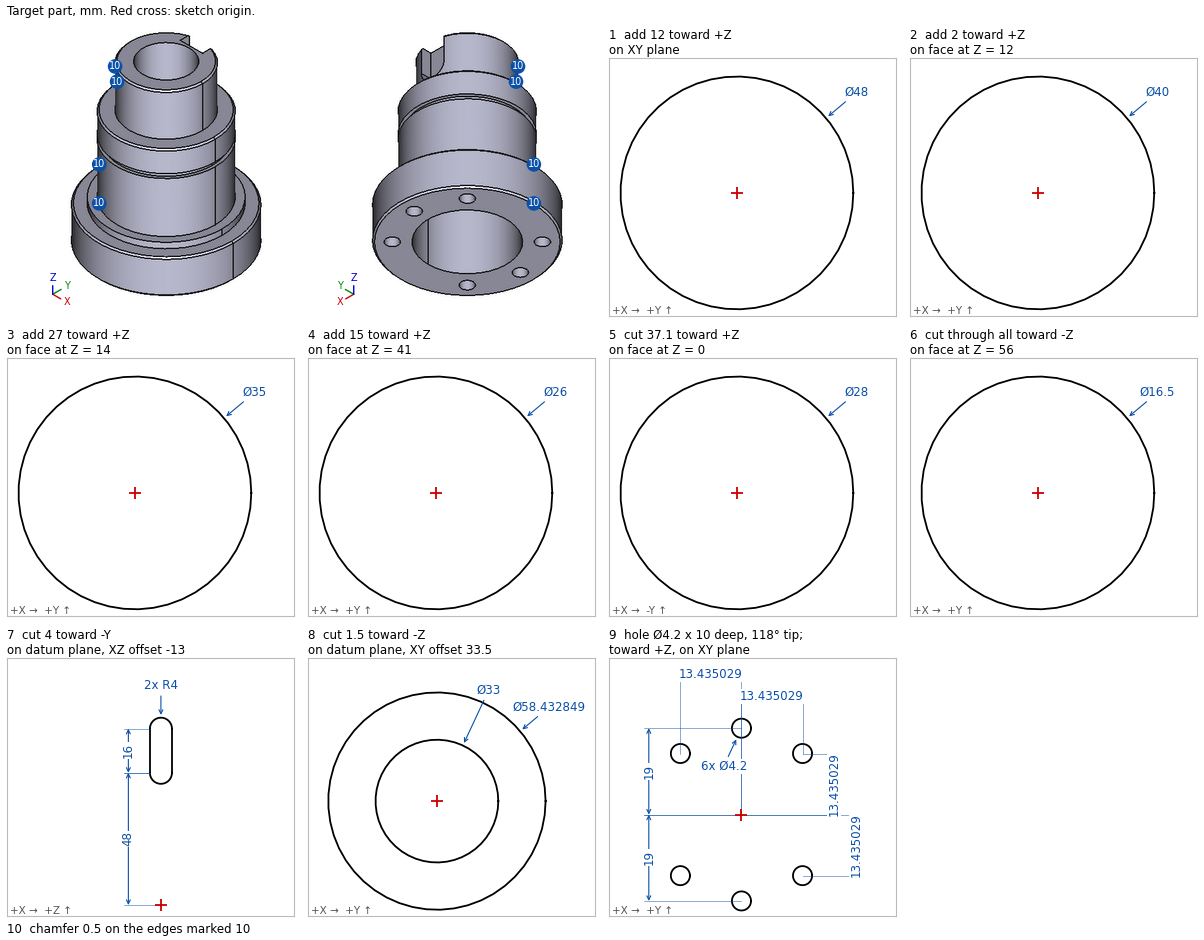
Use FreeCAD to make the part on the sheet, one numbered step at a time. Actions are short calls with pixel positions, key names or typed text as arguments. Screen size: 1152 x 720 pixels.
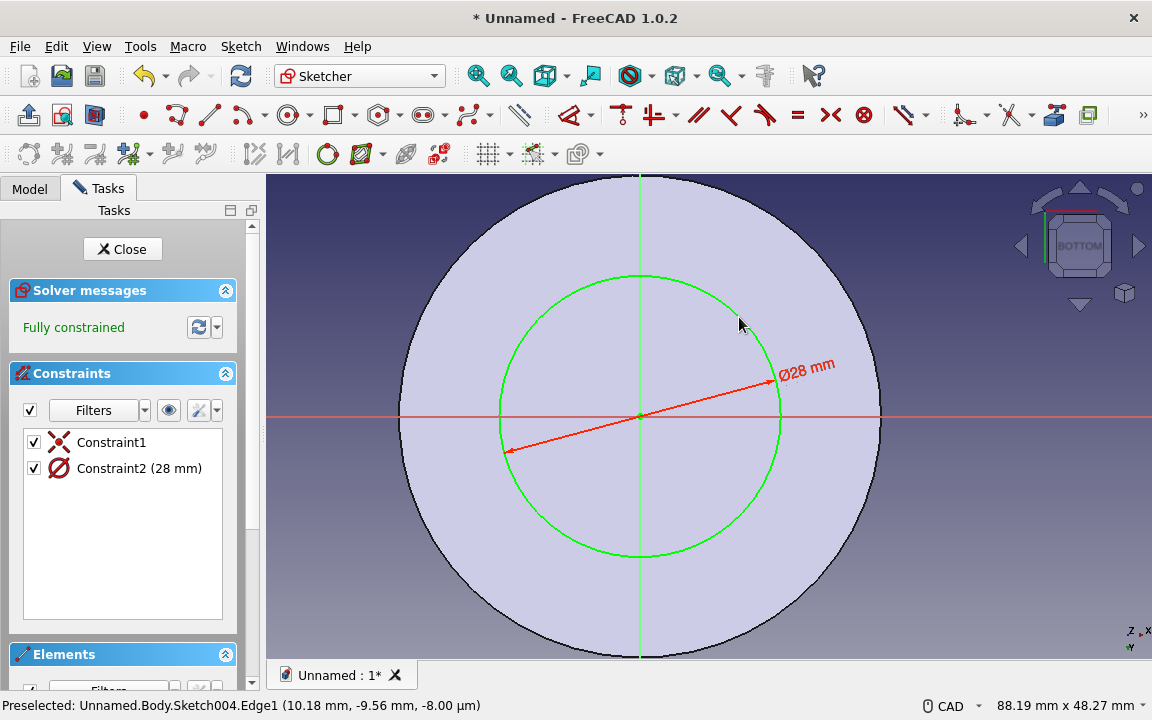
click(123, 249)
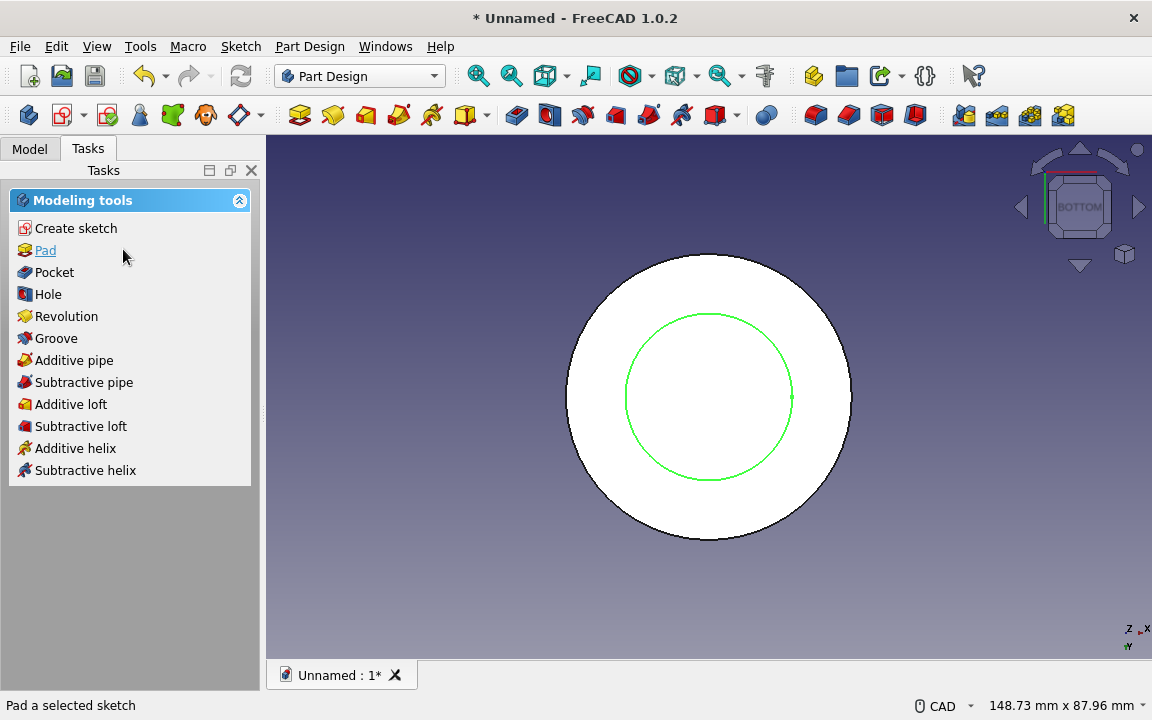
click(517, 116)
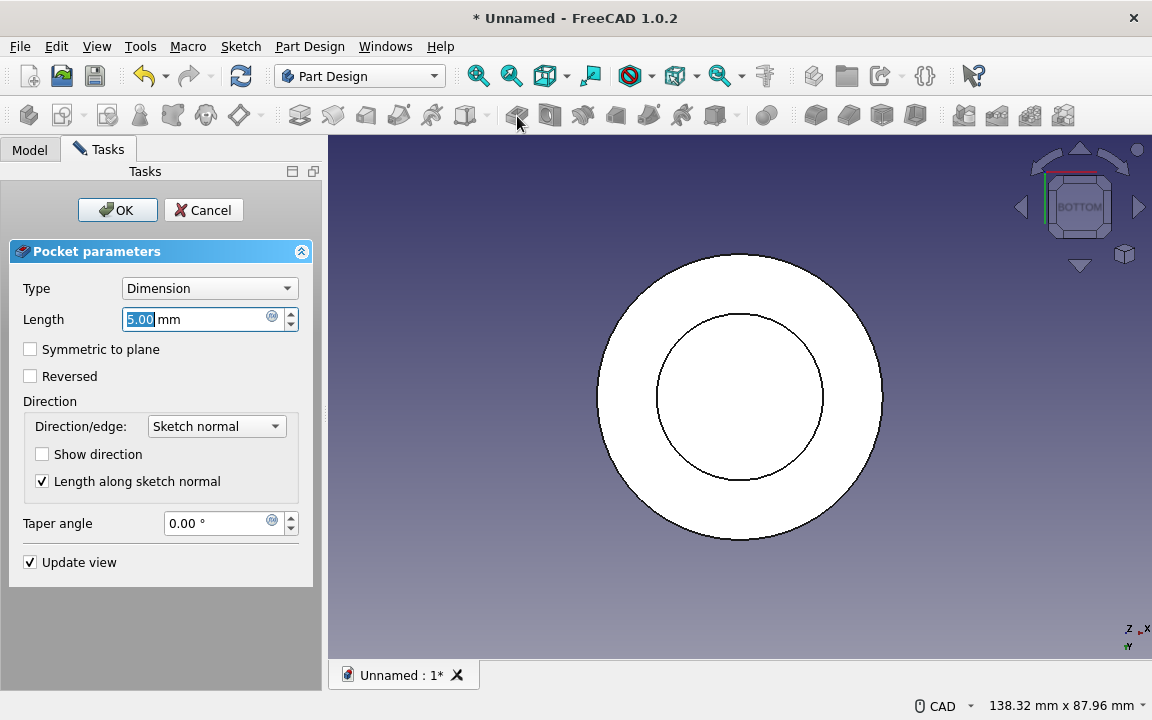
text(37.1)
key(Tab)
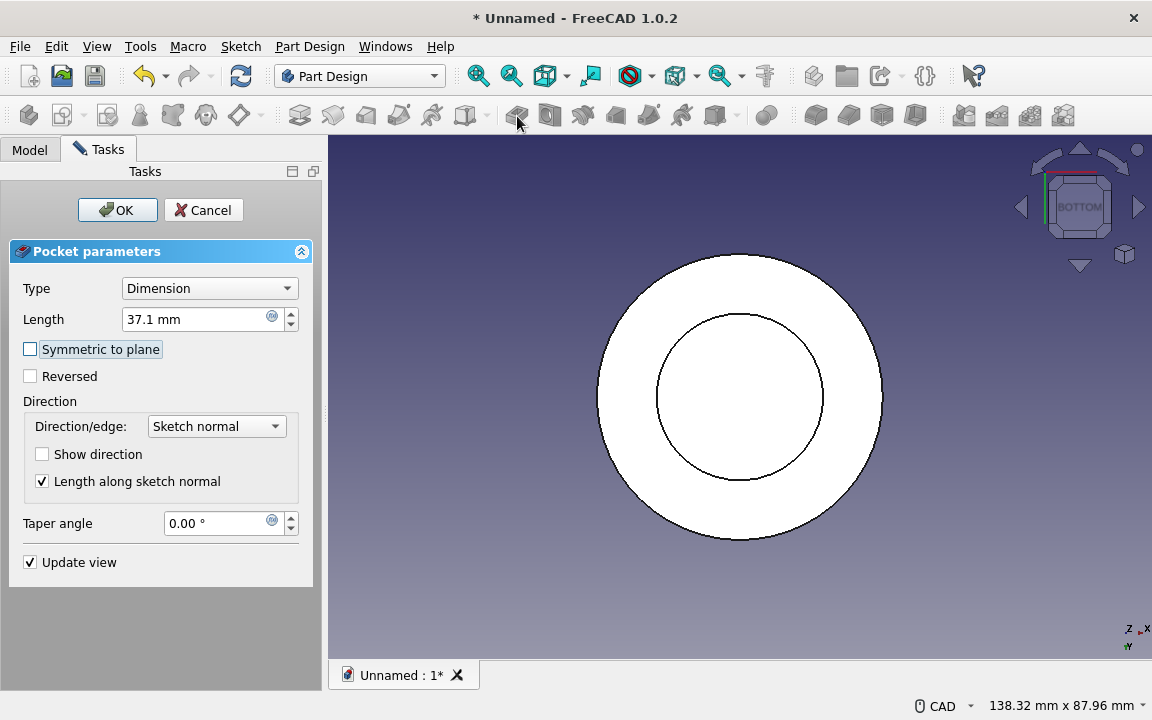
click(118, 210)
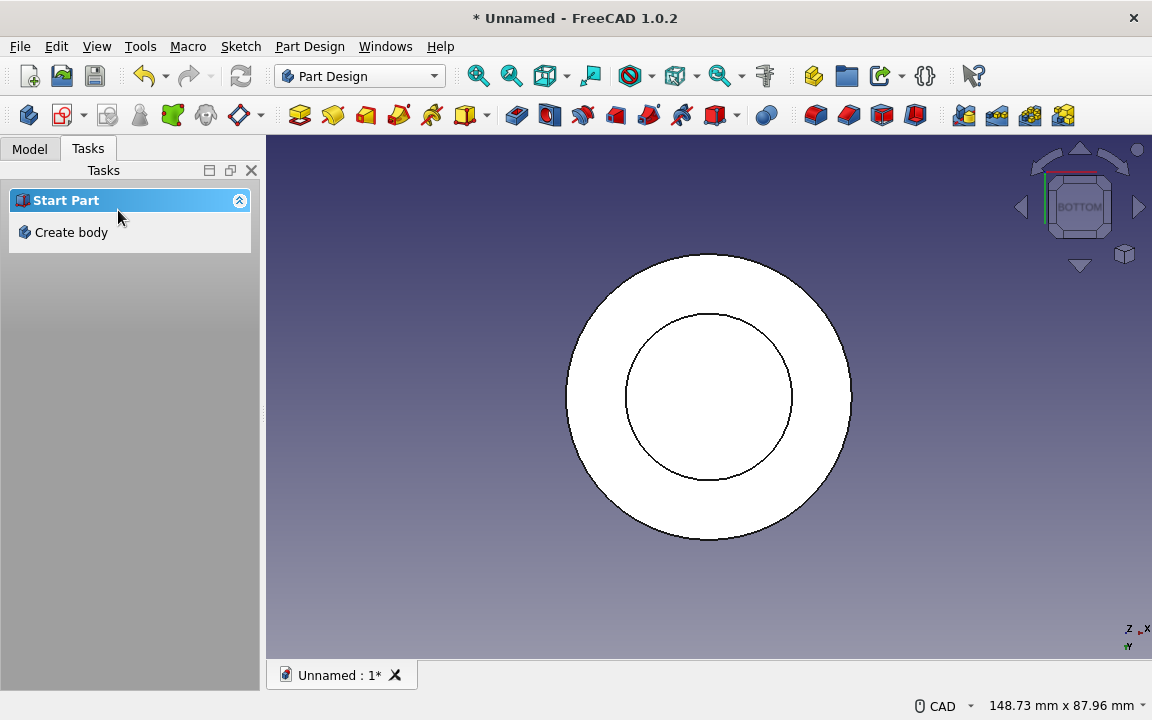
key(0)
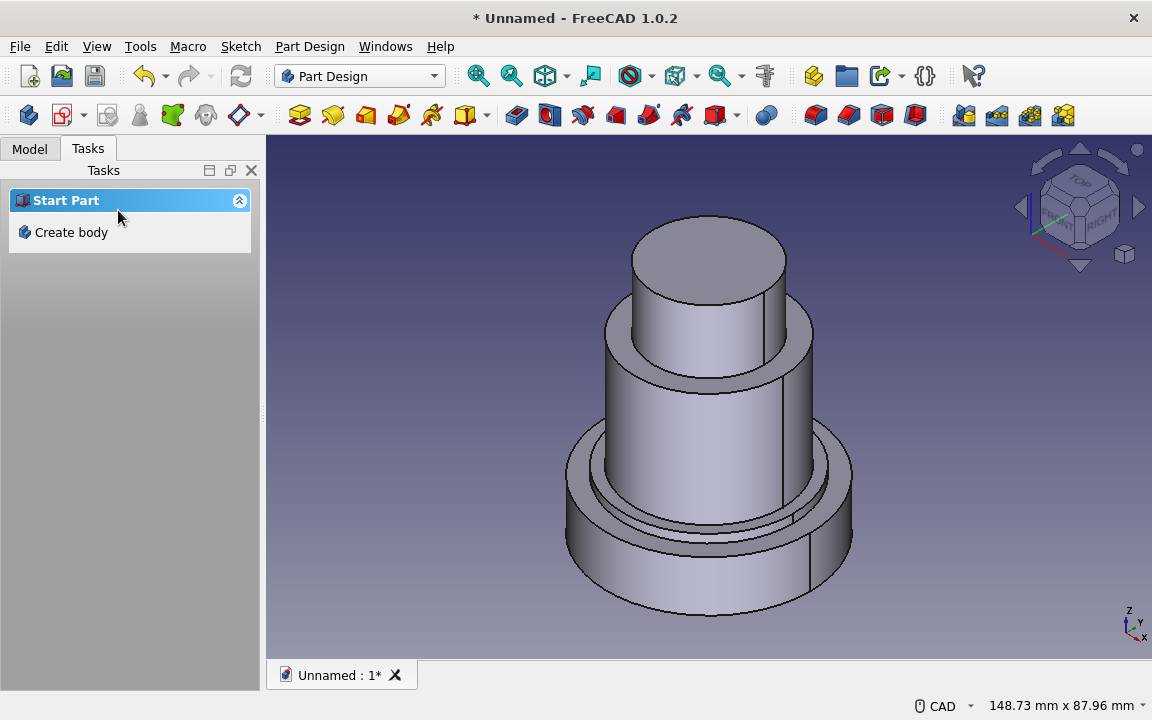
click(709, 260)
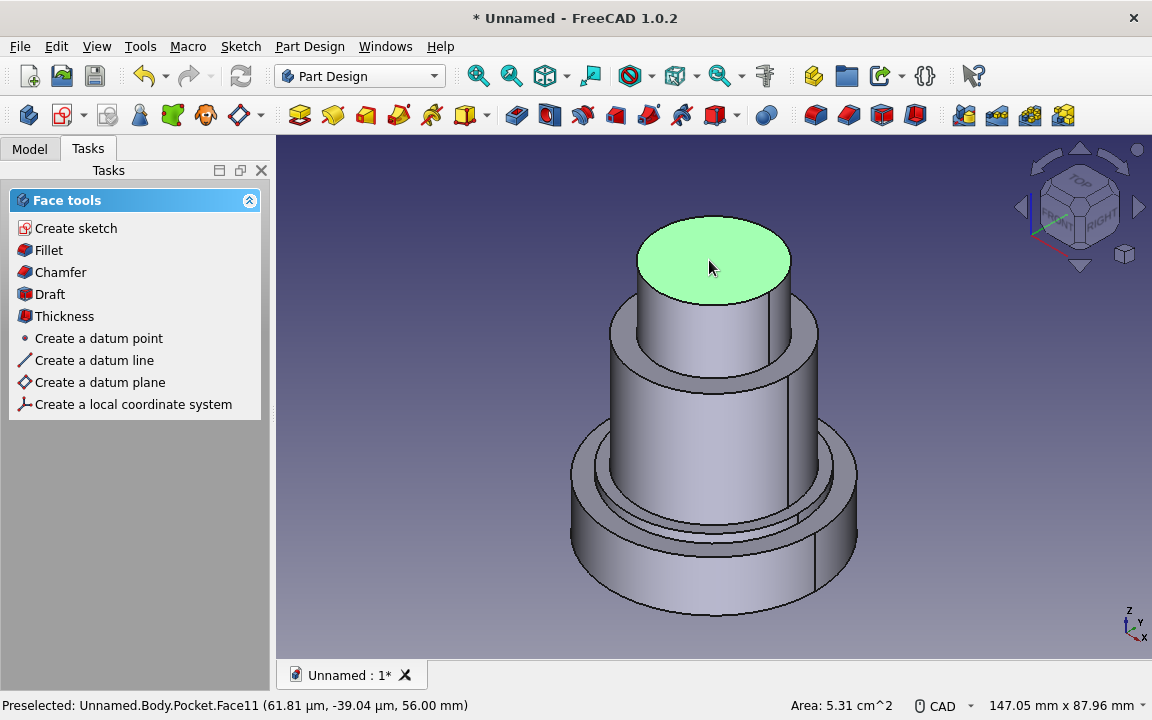
click(62, 116)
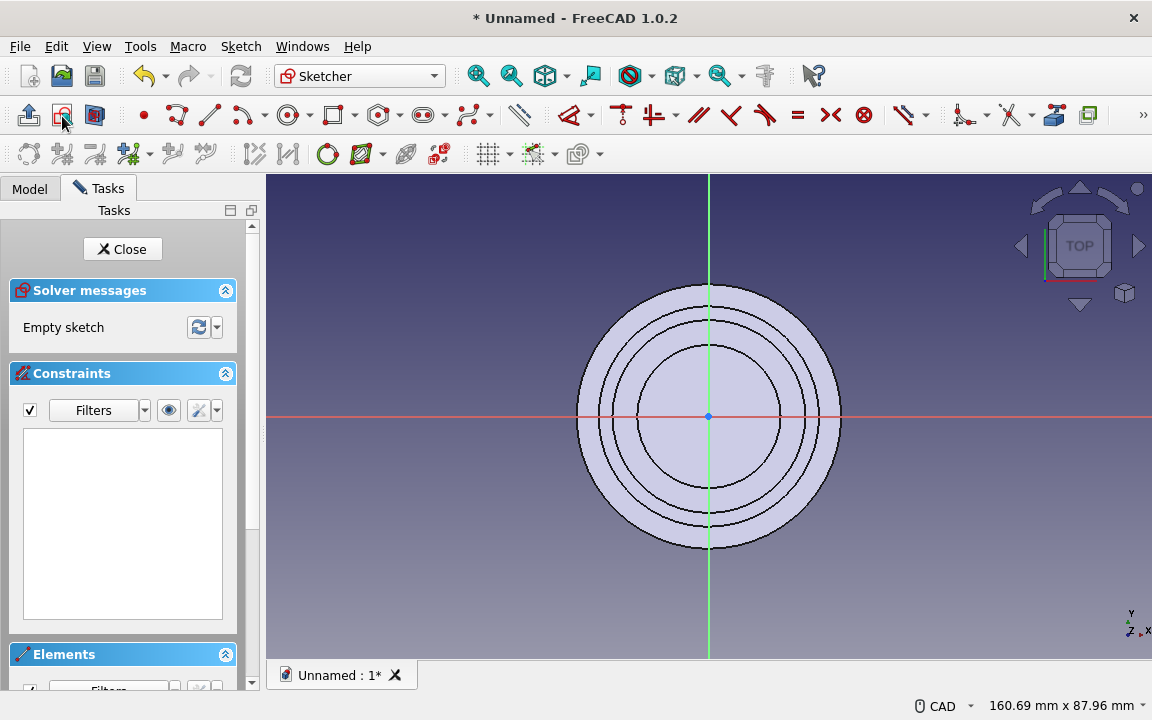
scroll(738, 416, up, 6)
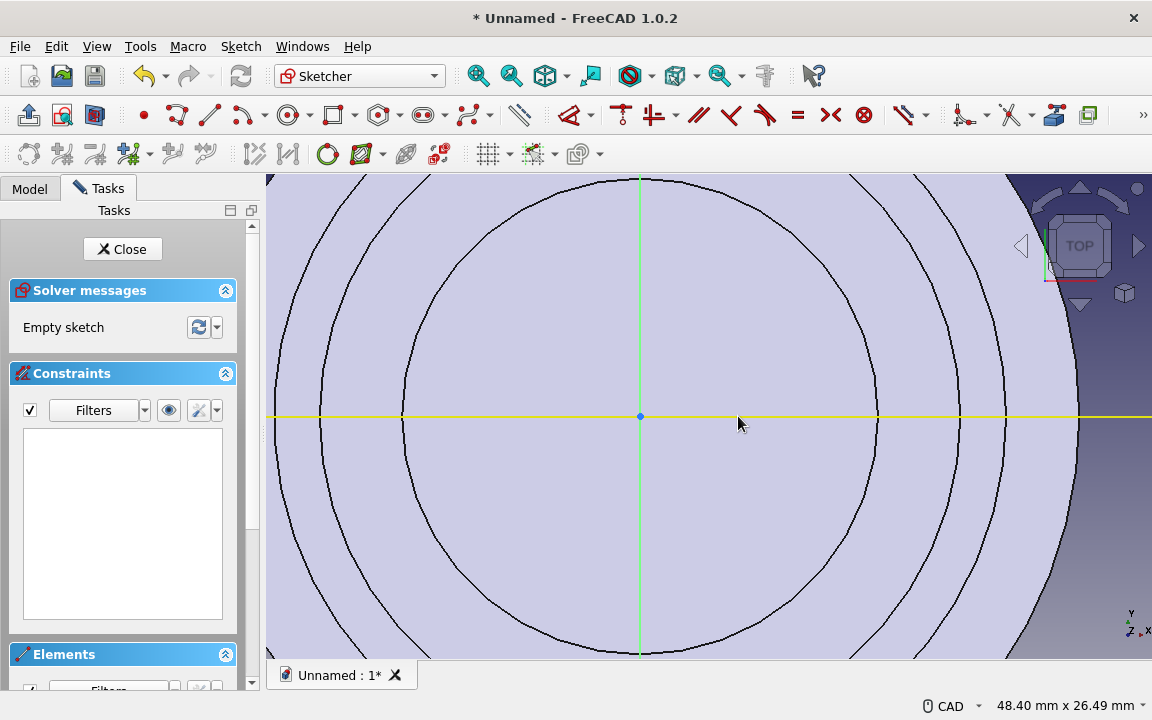
click(288, 116)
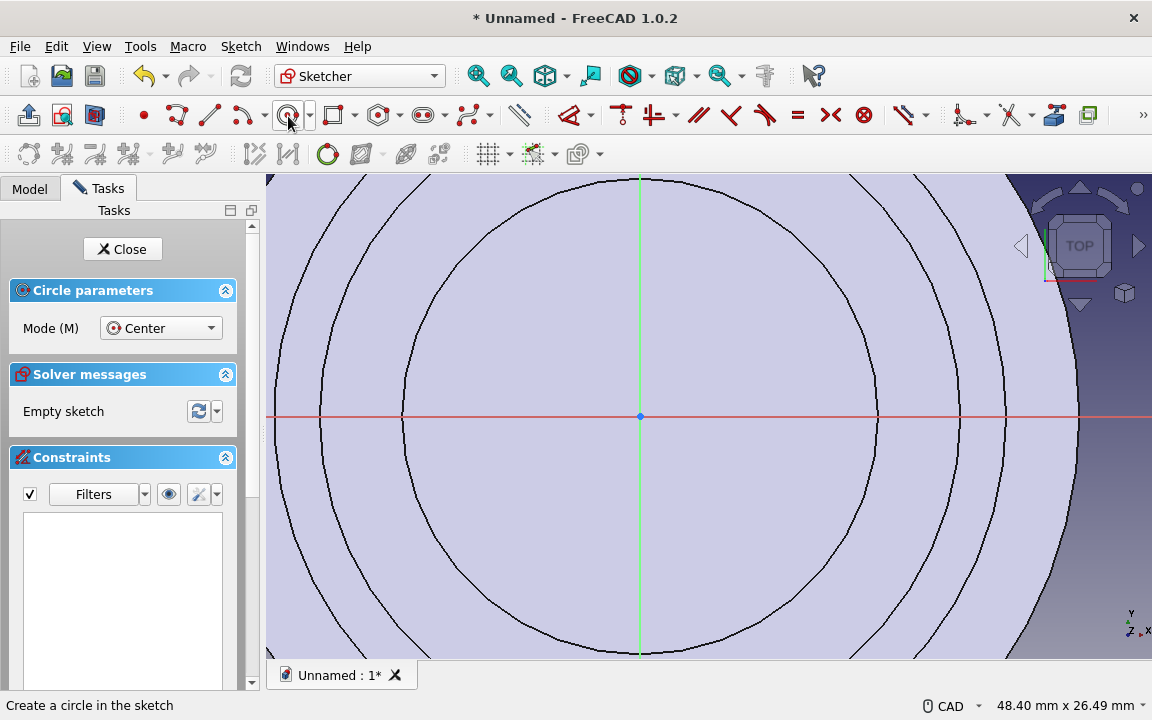
click(640, 416)
click(747, 310)
key(Escape)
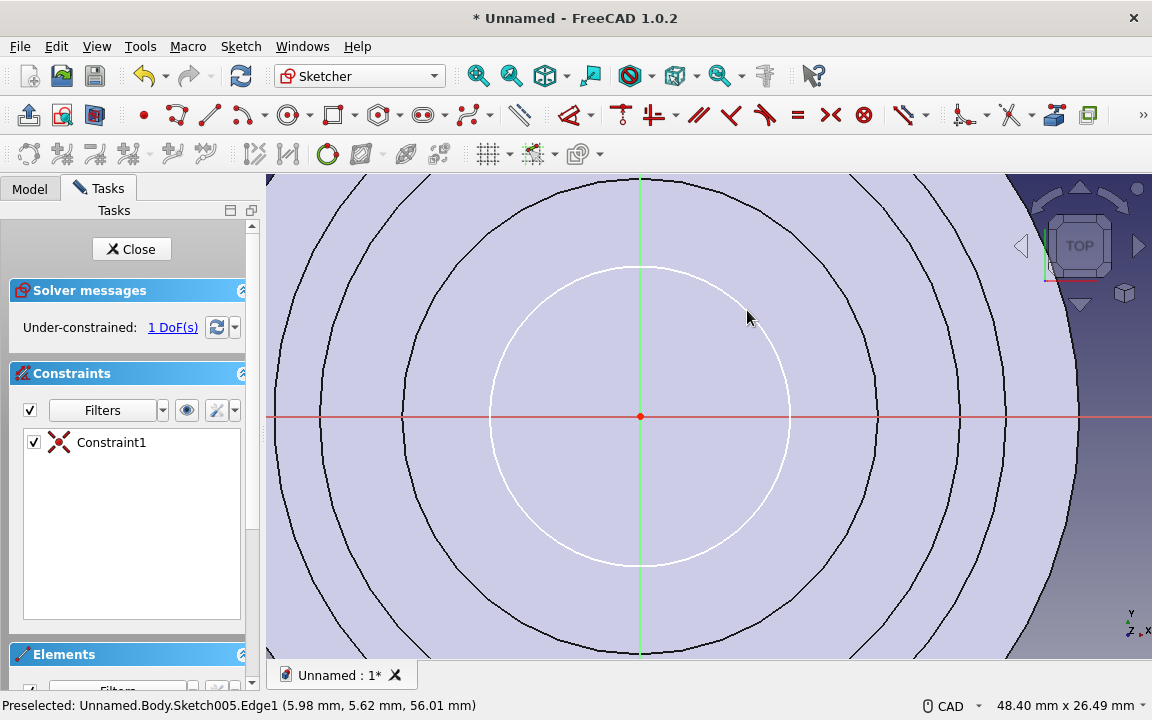
click(746, 310)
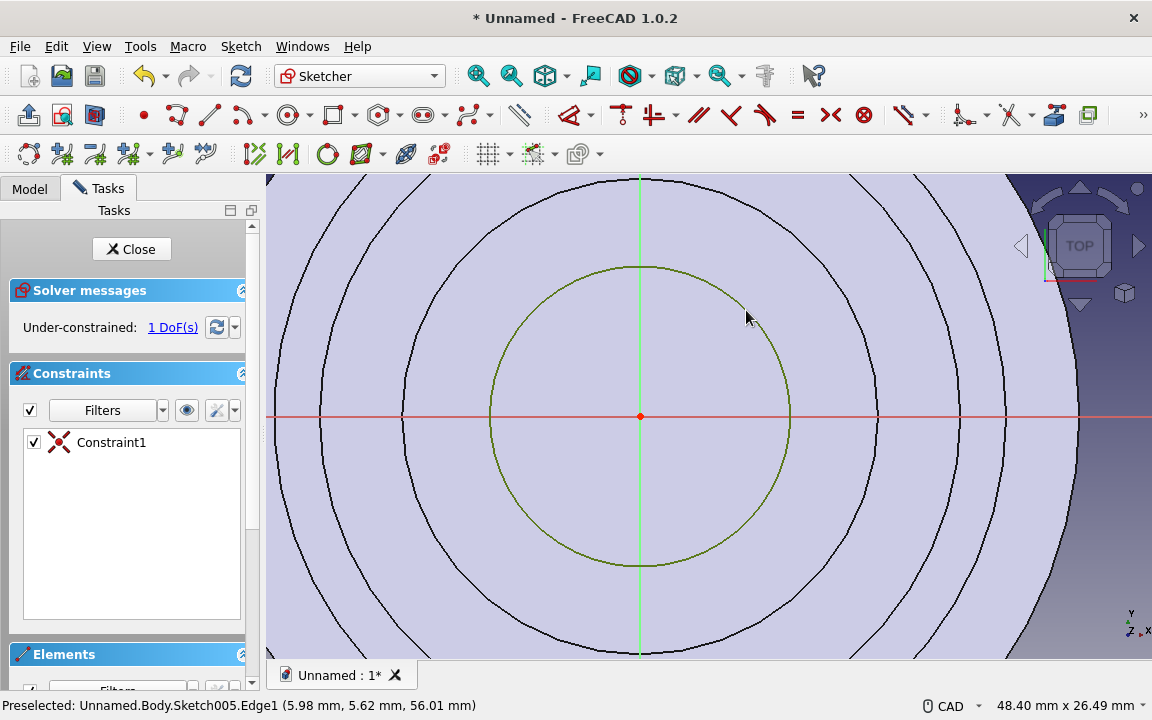
key(k)
key(o)